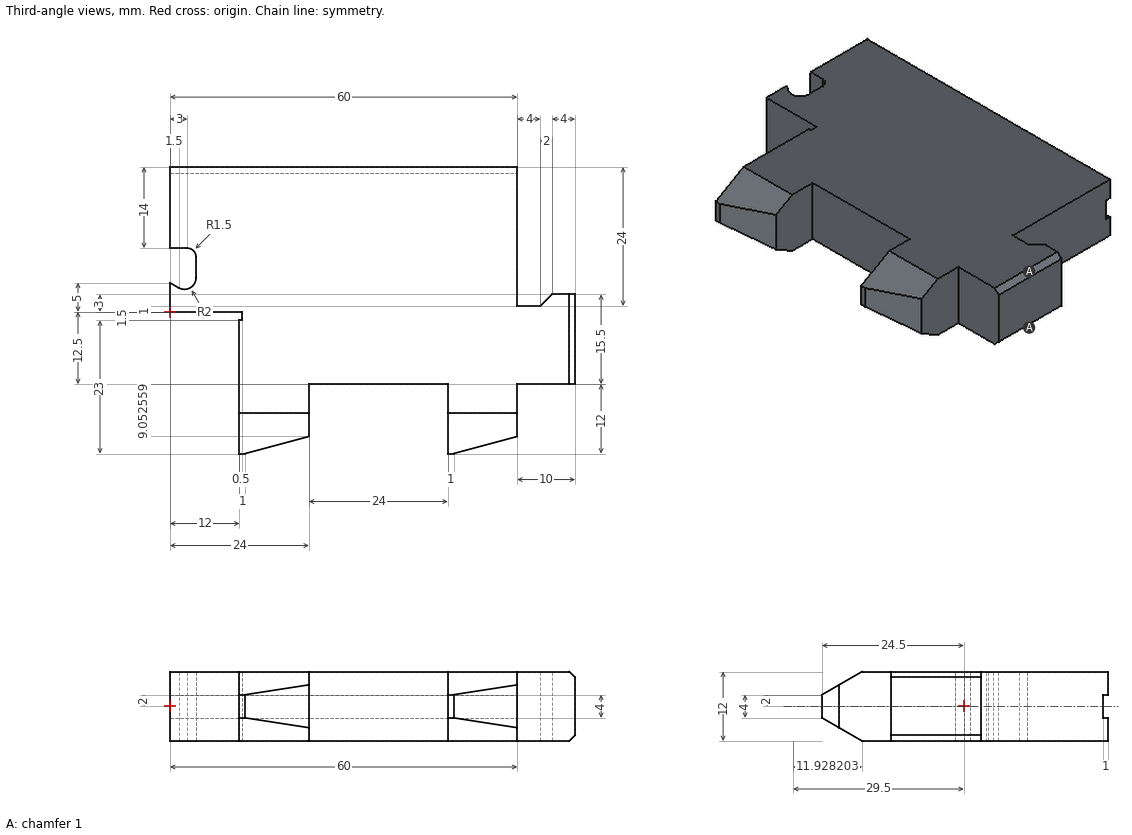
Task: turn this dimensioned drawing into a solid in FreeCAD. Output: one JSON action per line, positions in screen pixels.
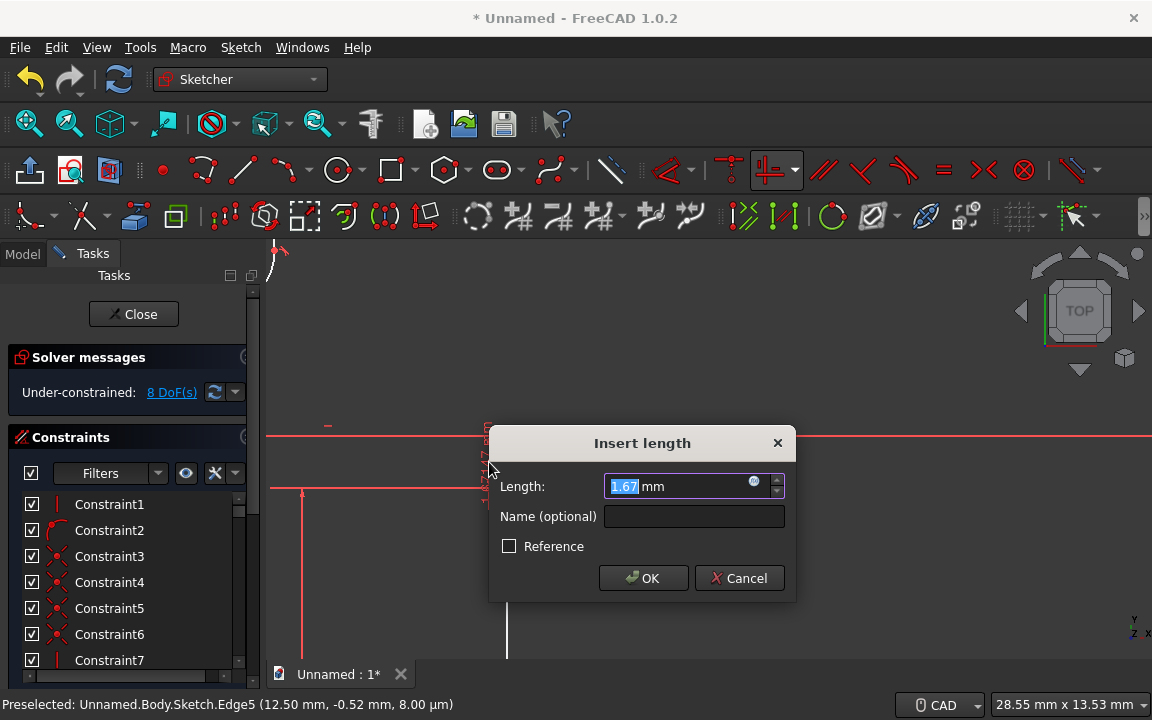
{"action": "type", "text": "1.5"}
{"action": "key", "text": "Return"}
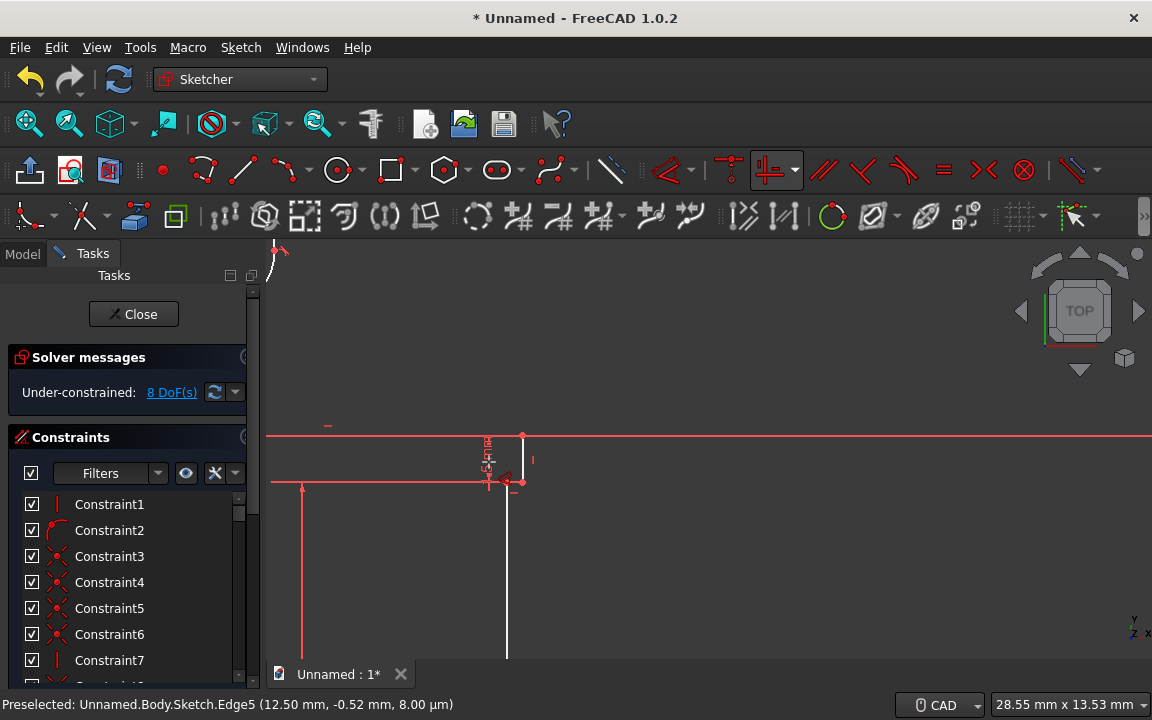
{"action": "scroll", "coordinate": [515, 482], "scroll_direction": "up", "scroll_amount": 5}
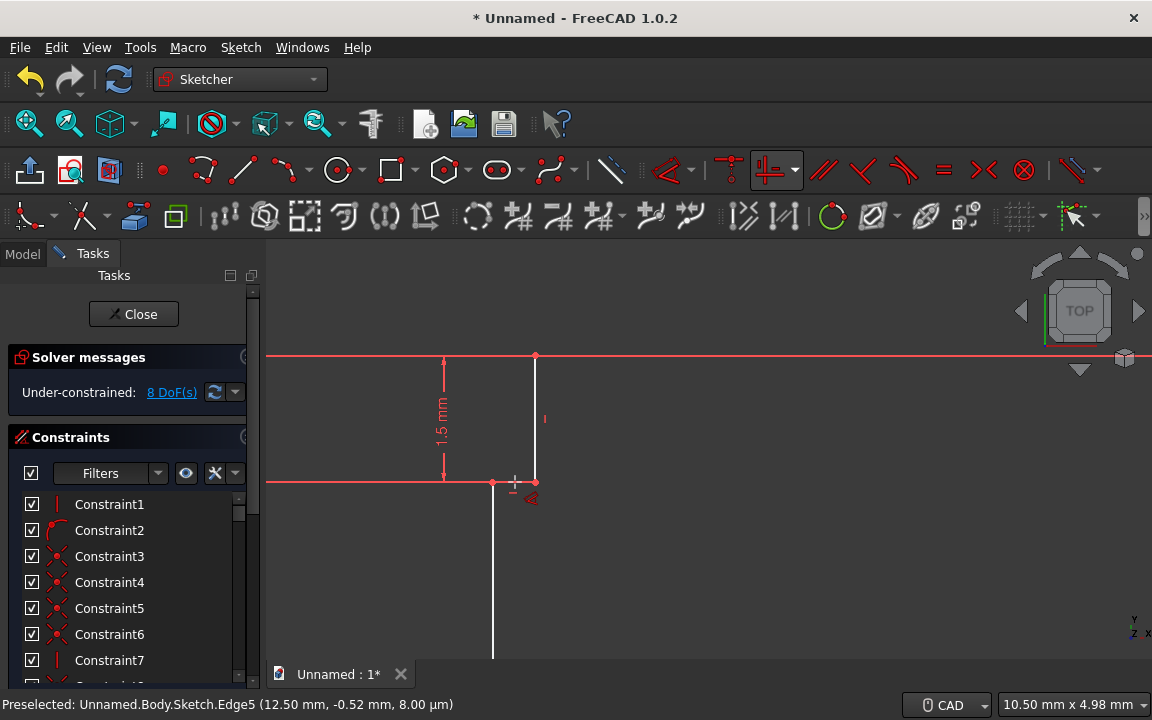
{"action": "left_click", "coordinate": [514, 482]}
{"action": "left_click", "coordinate": [514, 516]}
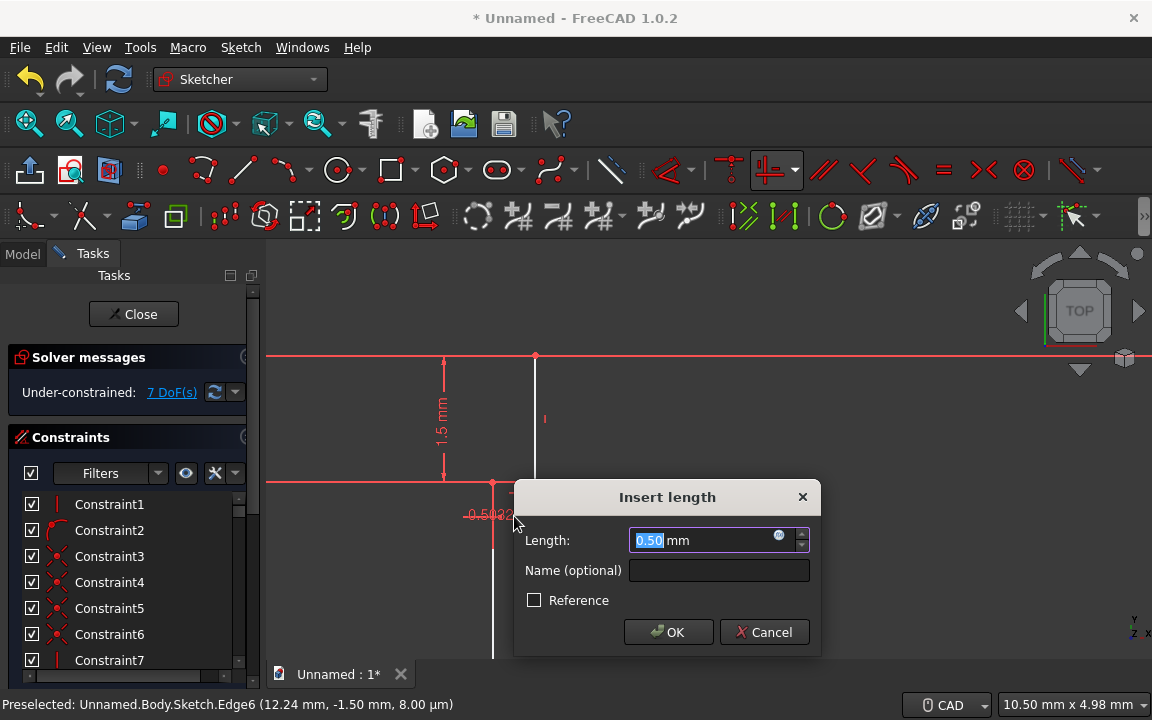
{"action": "type", "text": "0.5"}
{"action": "key", "text": "Return"}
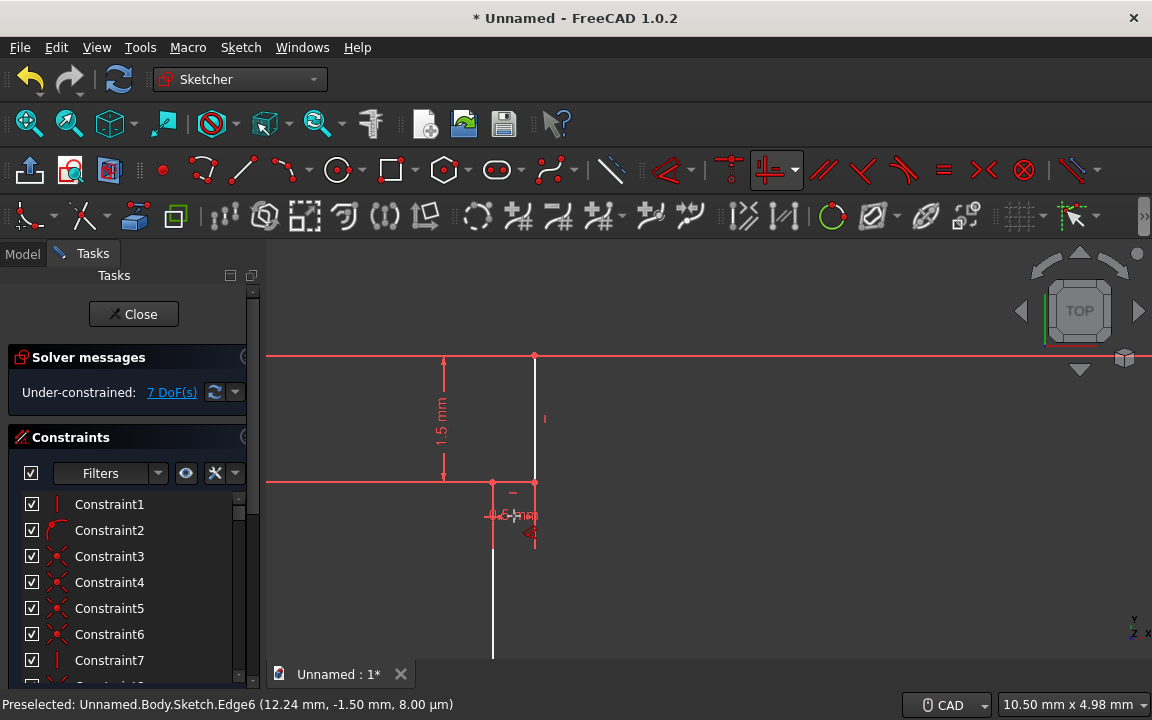
{"action": "scroll", "coordinate": [524, 456], "scroll_direction": "down", "scroll_amount": 14}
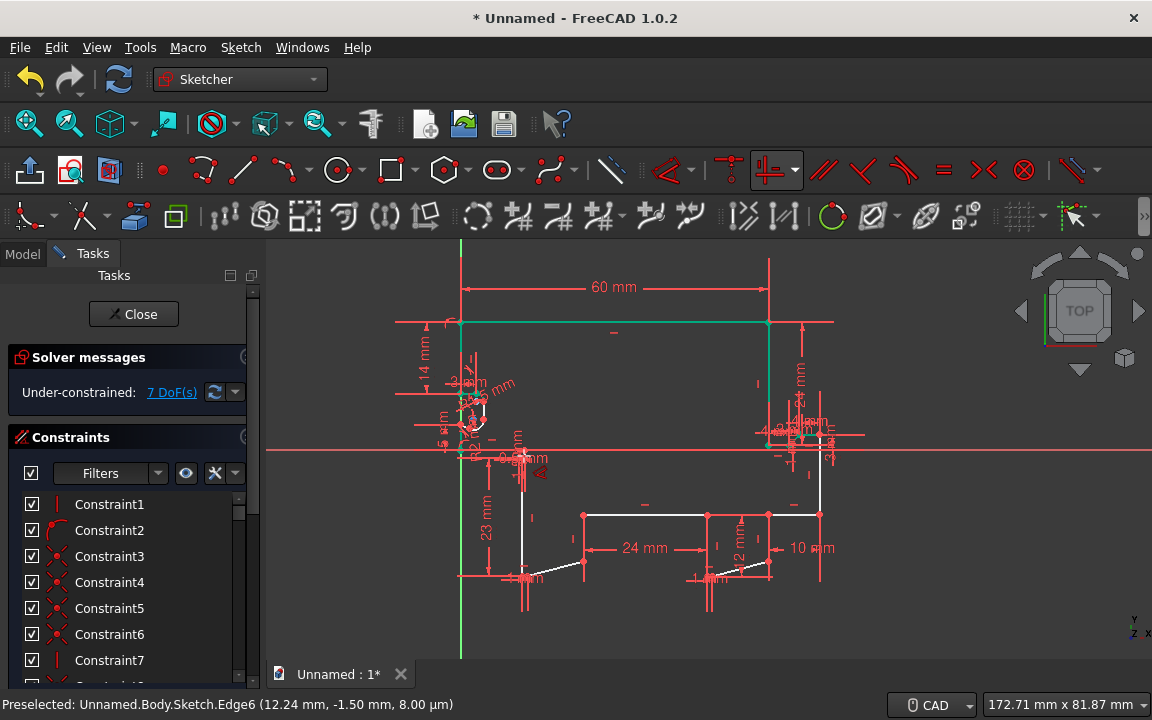
{"action": "scroll", "coordinate": [522, 458], "scroll_direction": "up", "scroll_amount": 8}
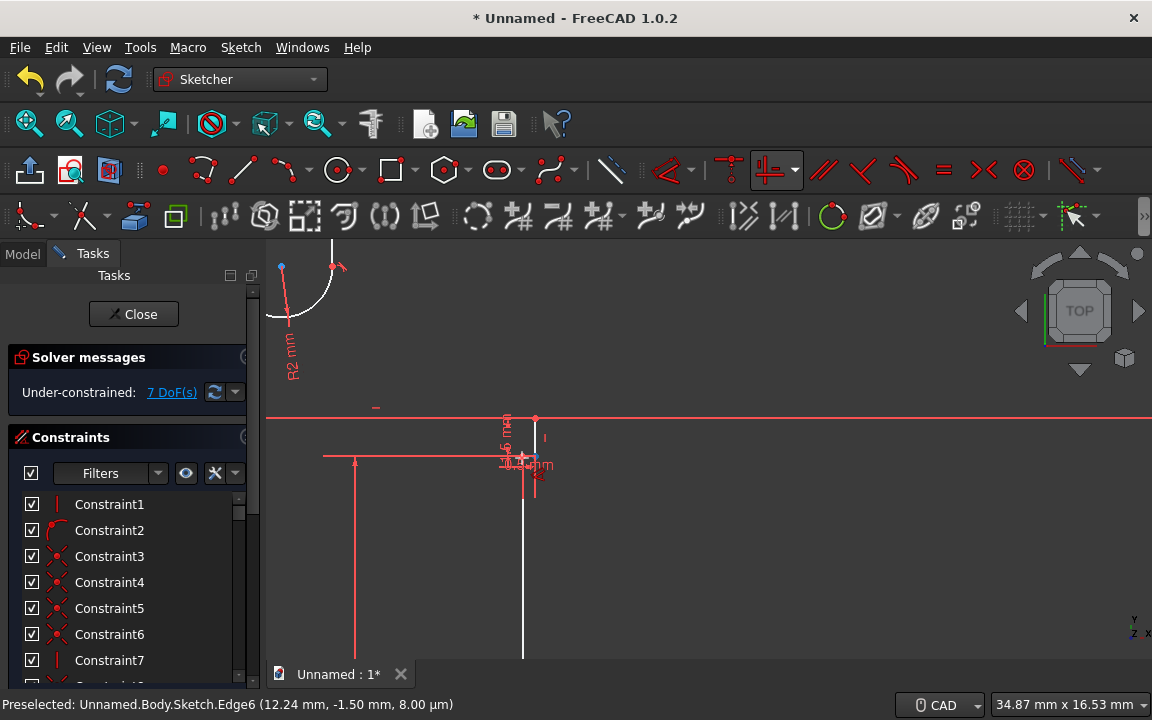
{"action": "left_click", "coordinate": [523, 456]}
{"action": "left_click", "coordinate": [408, 490]}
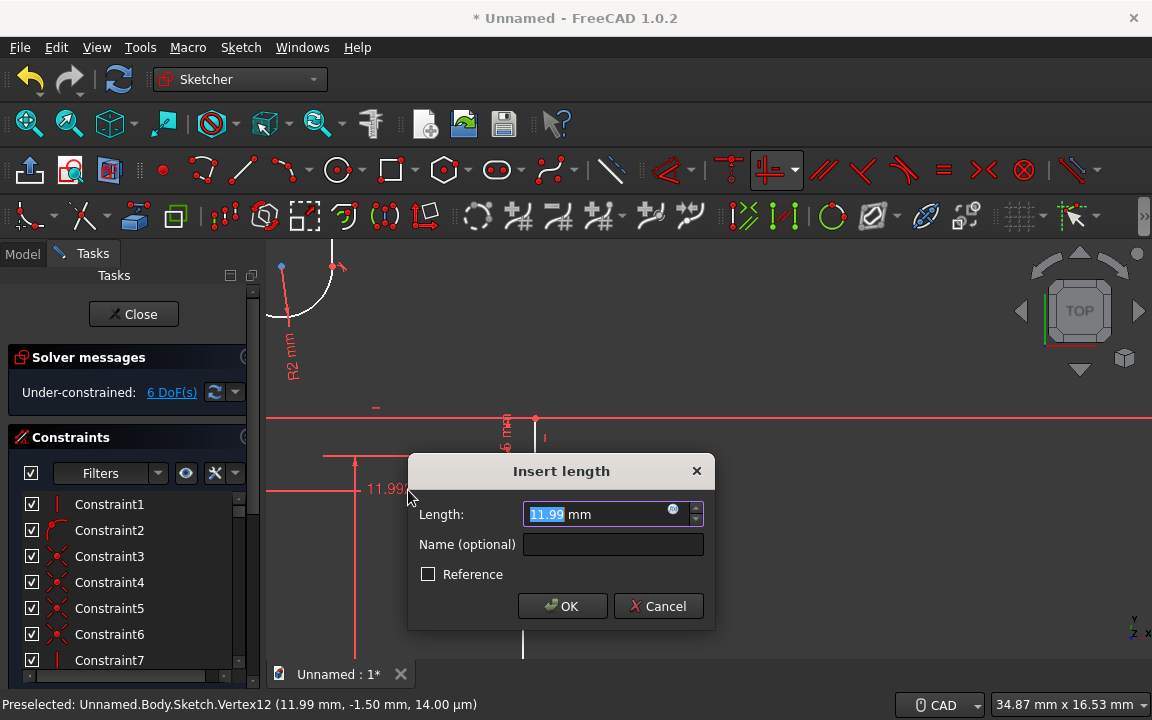
{"action": "type", "text": "12"}
{"action": "key", "text": "Return"}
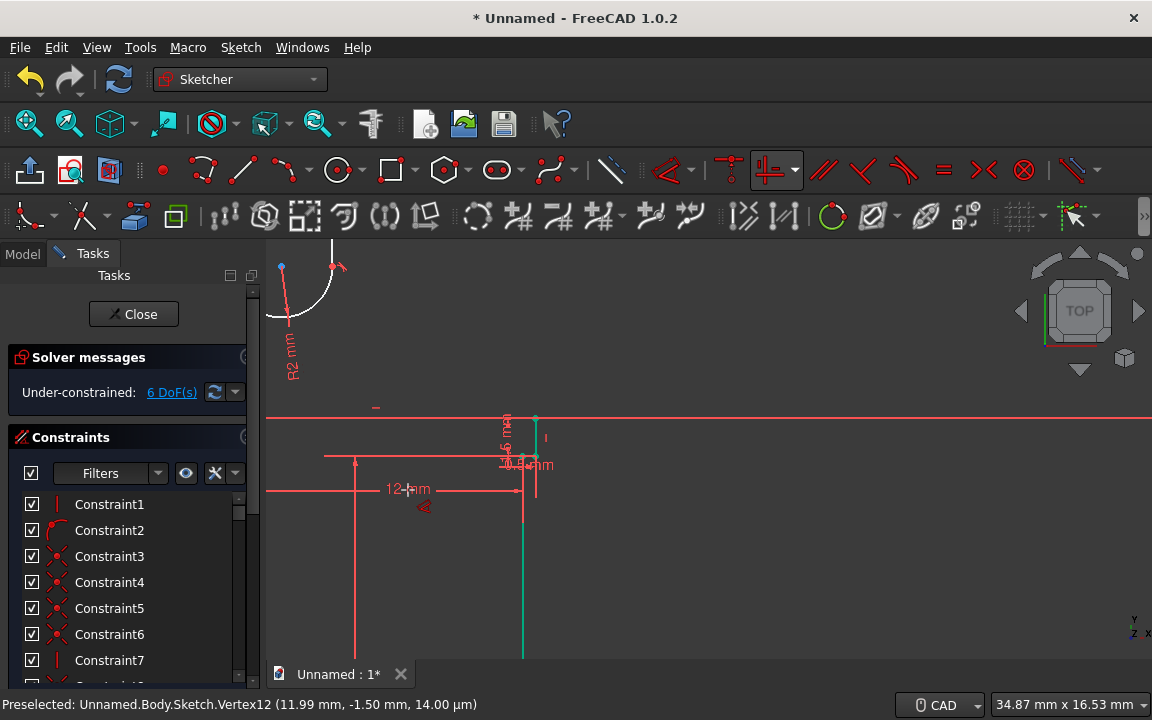
{"action": "scroll", "coordinate": [522, 458], "scroll_direction": "down", "scroll_amount": 8}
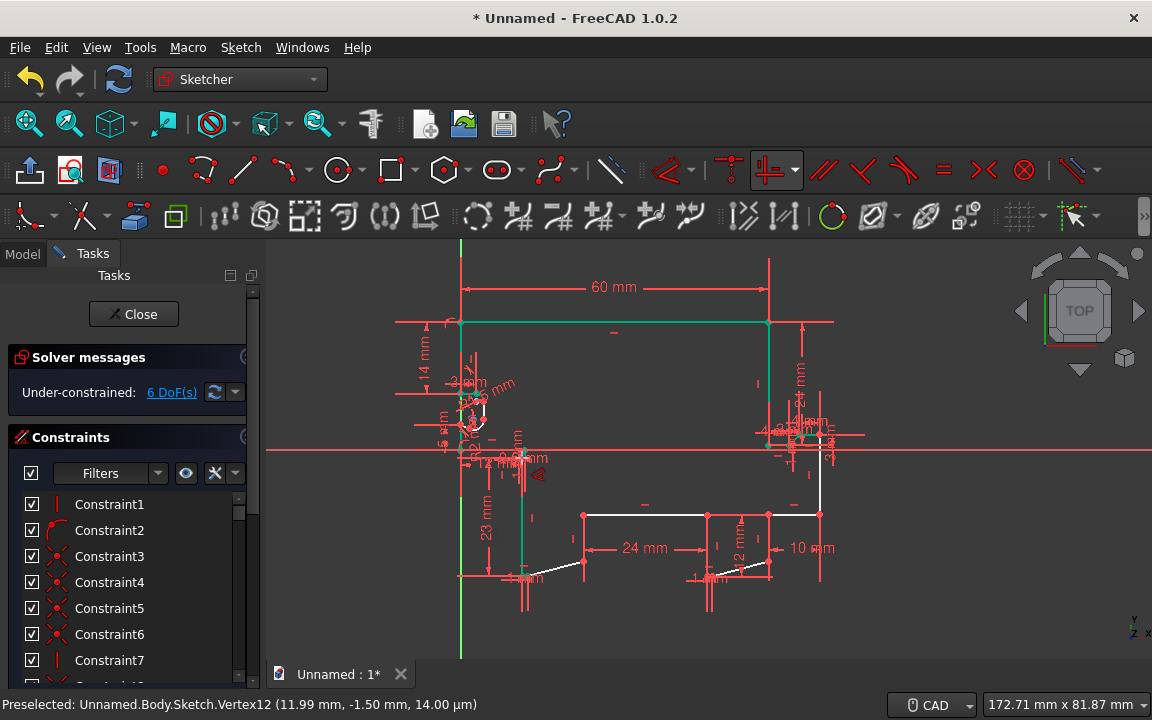
{"action": "left_click", "coordinate": [584, 561]}
{"action": "left_click", "coordinate": [565, 416]}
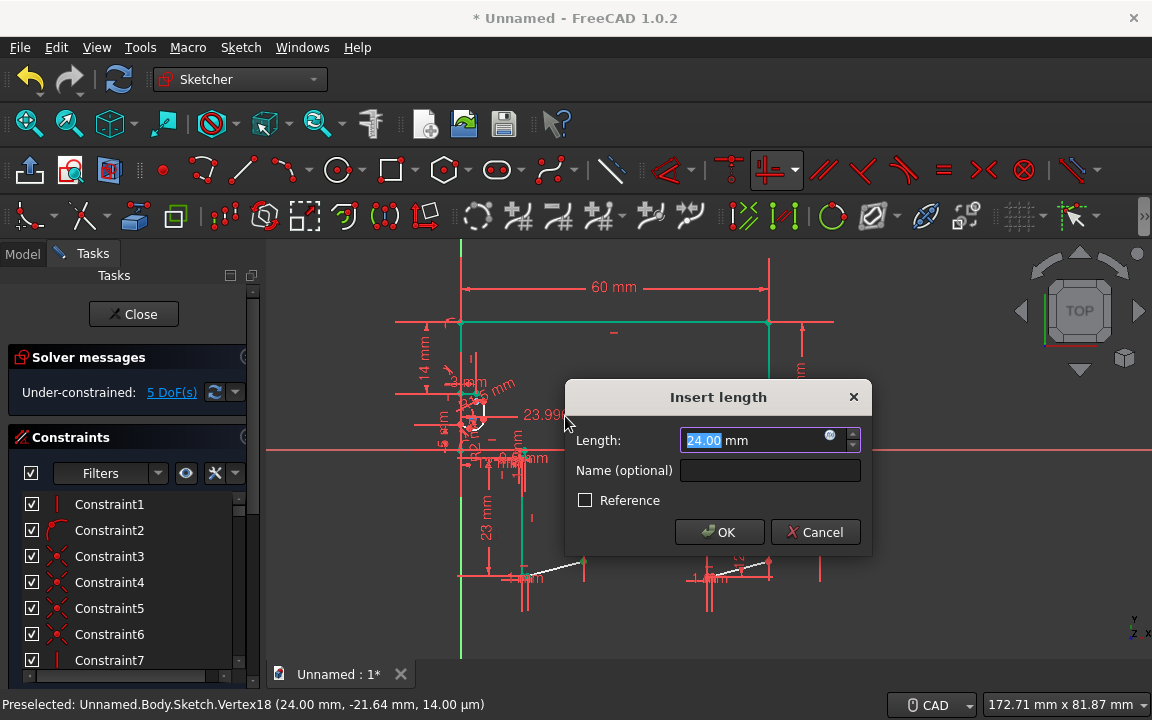
{"action": "type", "text": "24"}
{"action": "key", "text": "Return"}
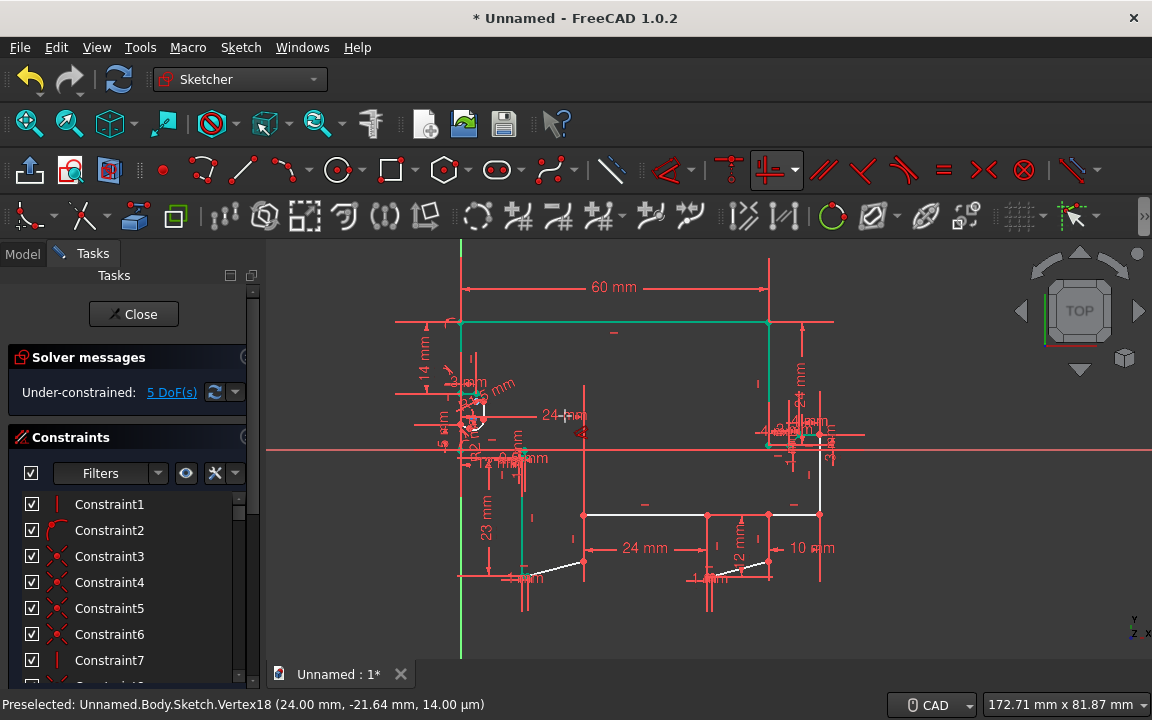
{"action": "left_click", "coordinate": [820, 491]}
{"action": "left_click", "coordinate": [854, 475]}